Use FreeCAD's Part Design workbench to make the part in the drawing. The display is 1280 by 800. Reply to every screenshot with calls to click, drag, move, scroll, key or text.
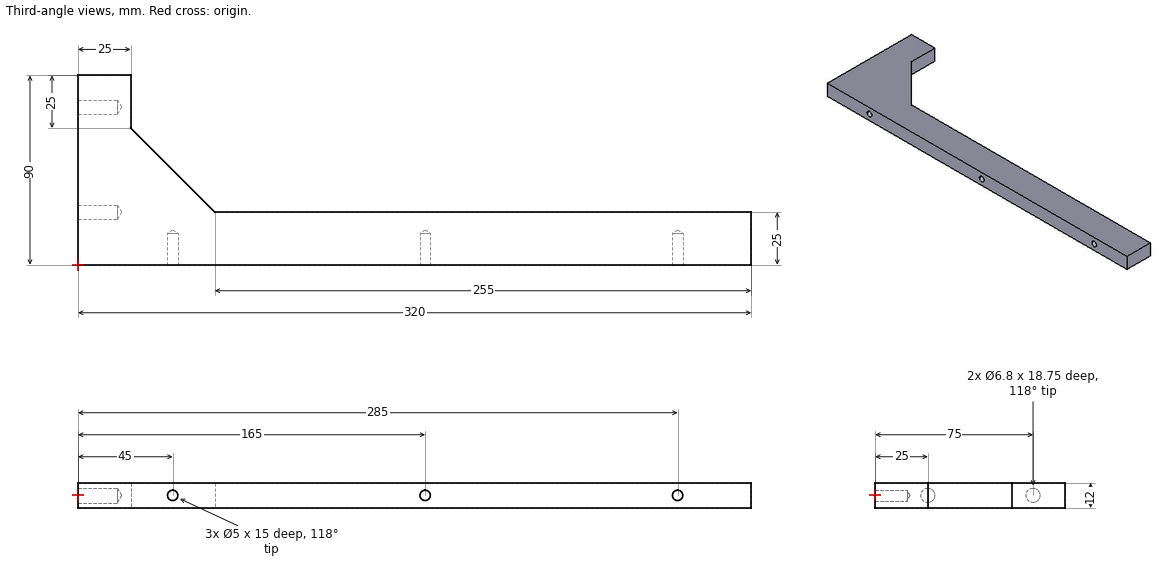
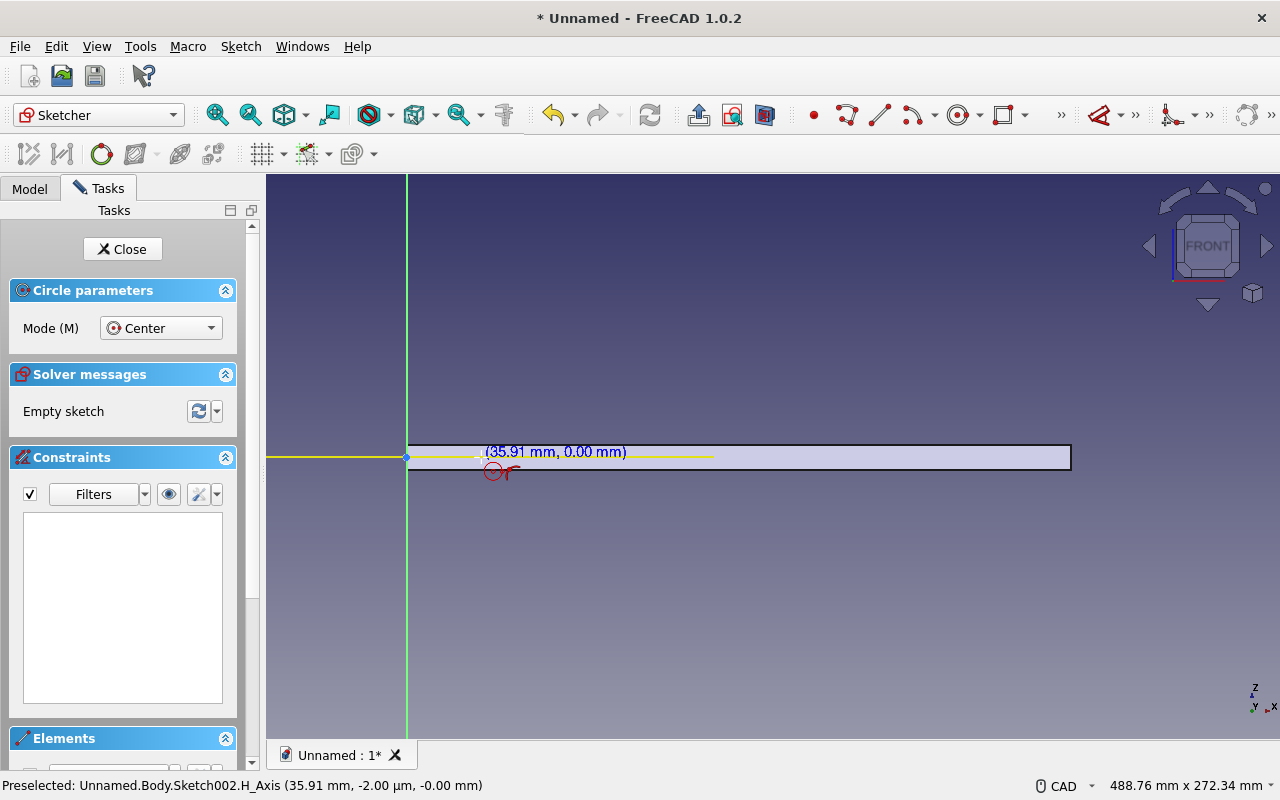
click(500, 457)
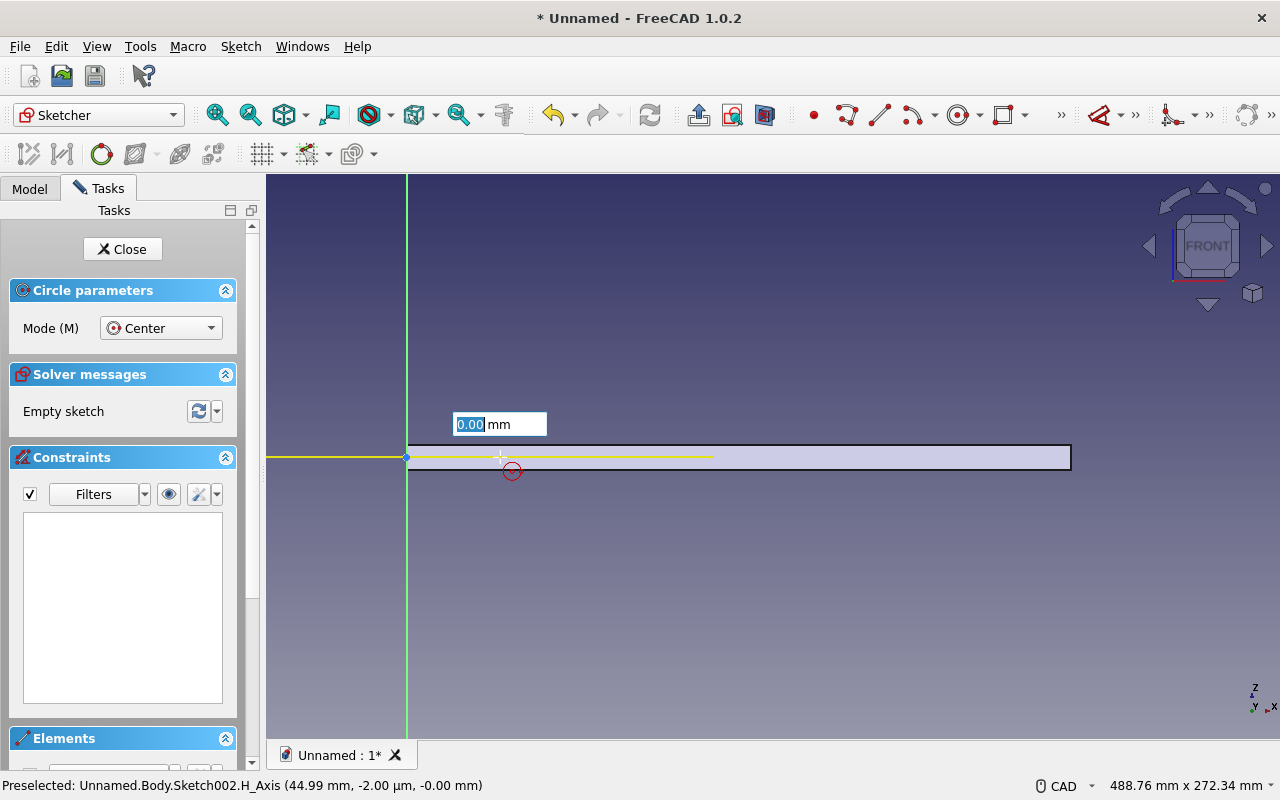
scroll(498, 462, up, 6)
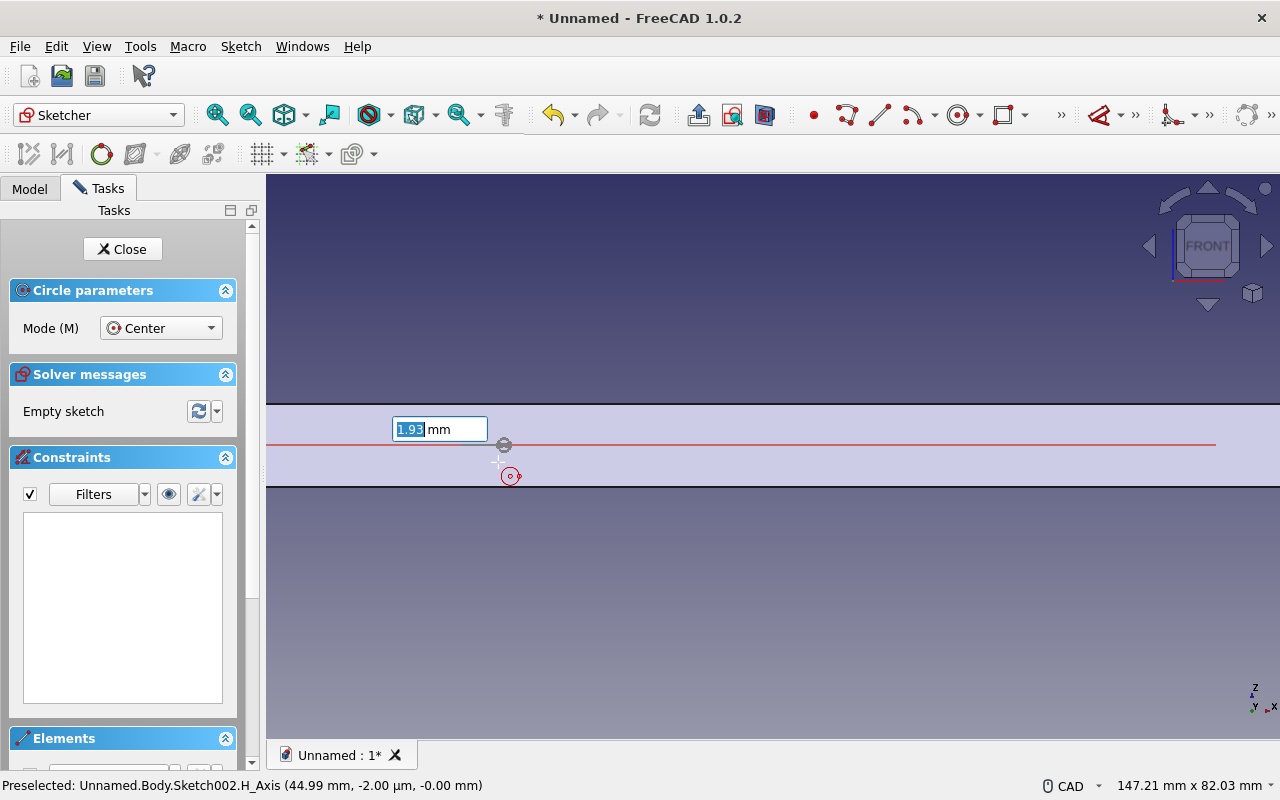
click(498, 461)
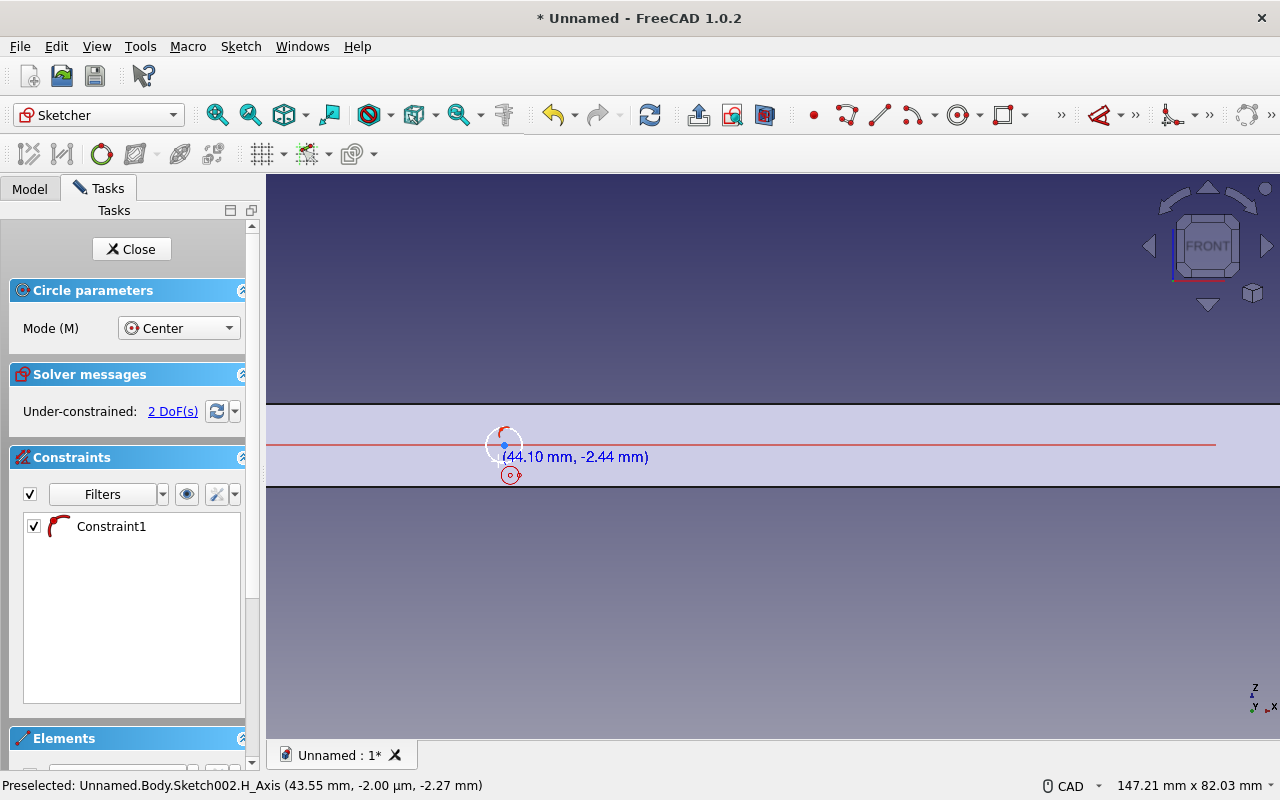
scroll(498, 461, down, 6)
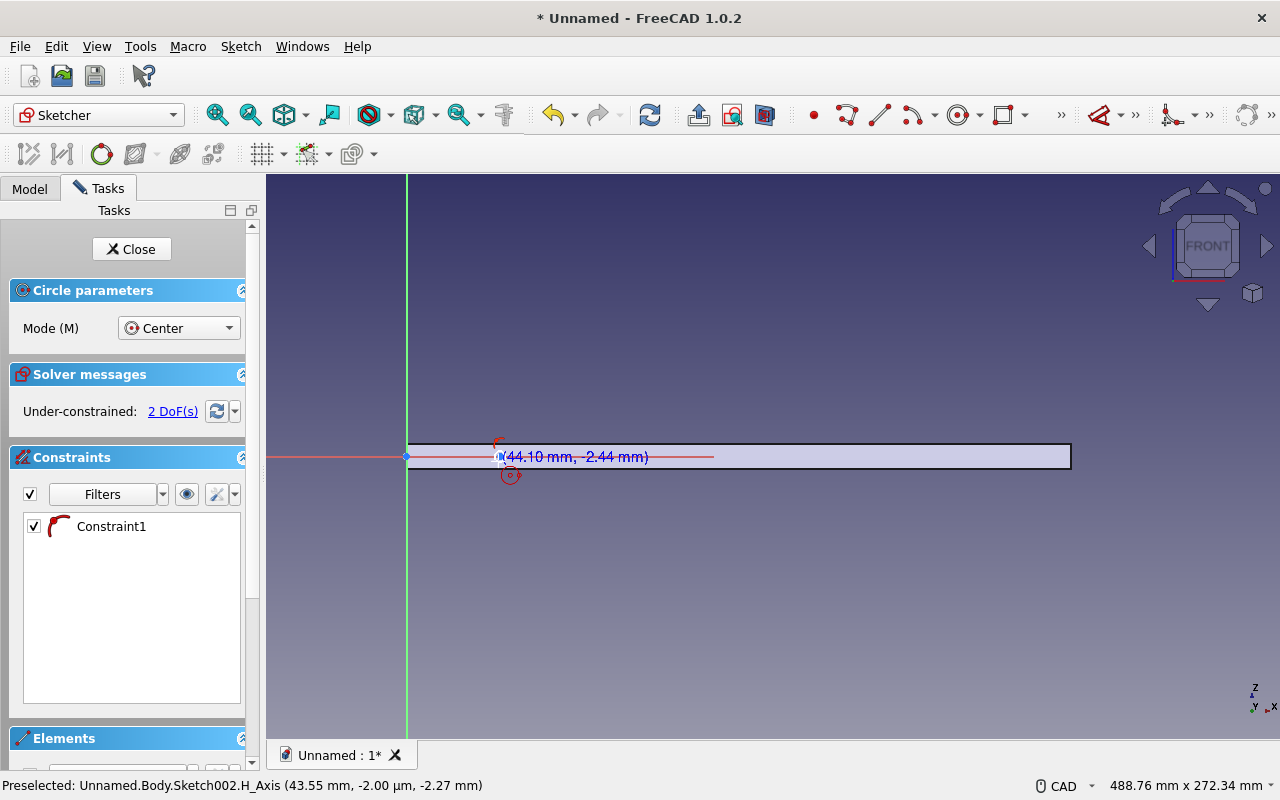
scroll(749, 457, up, 8)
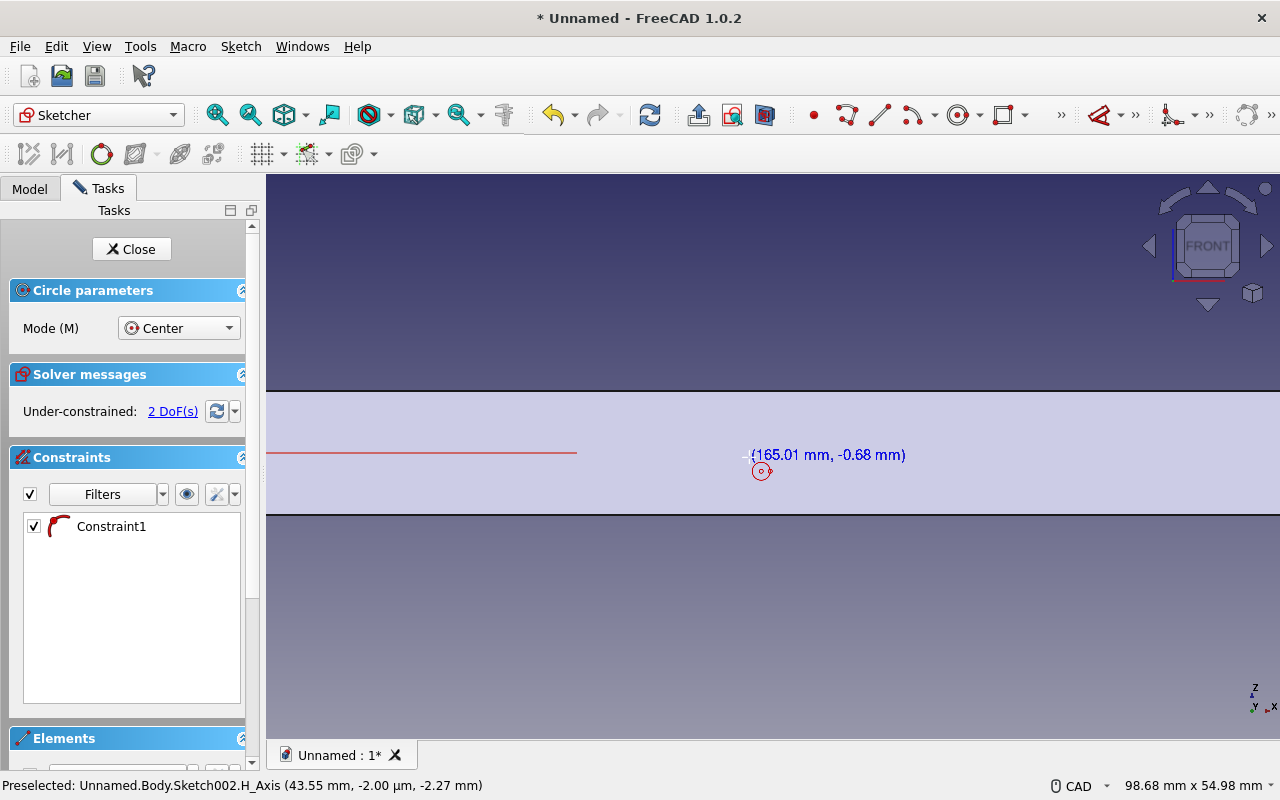
scroll(749, 457, down, 8)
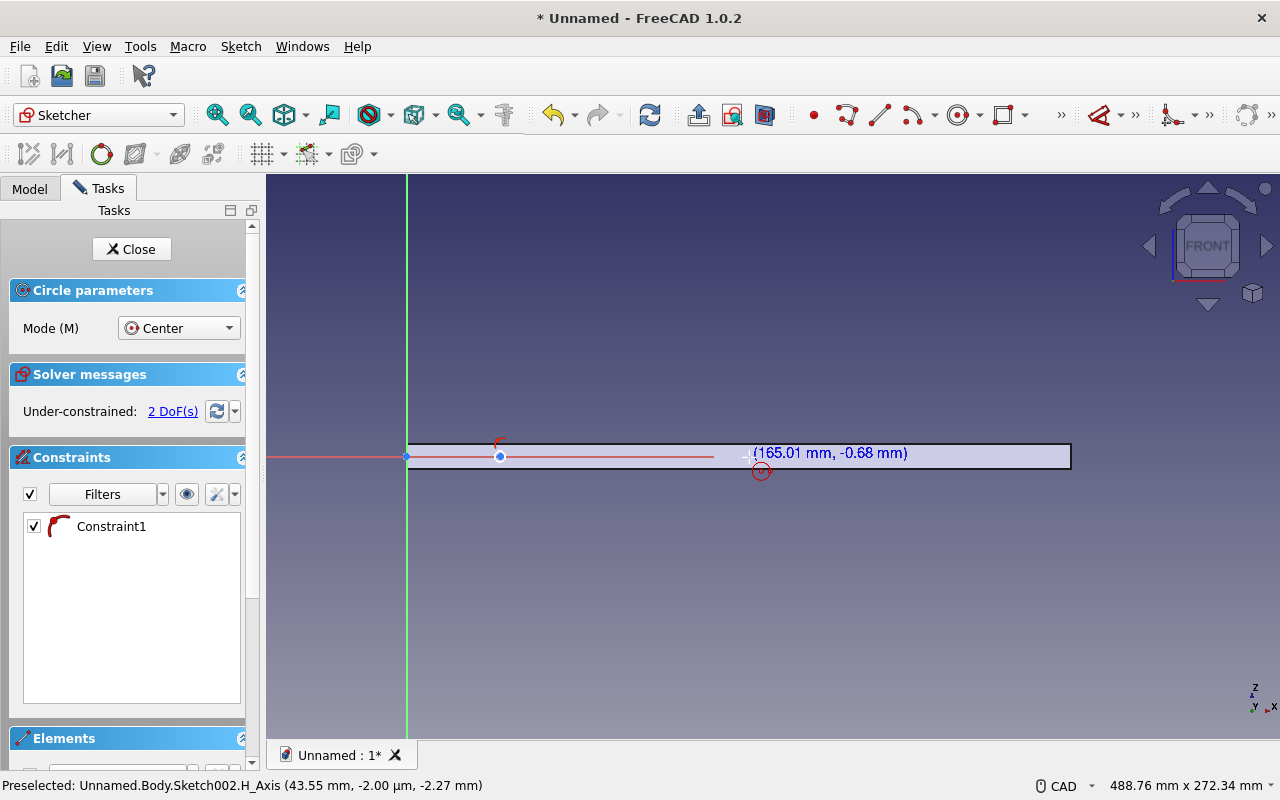
click(749, 457)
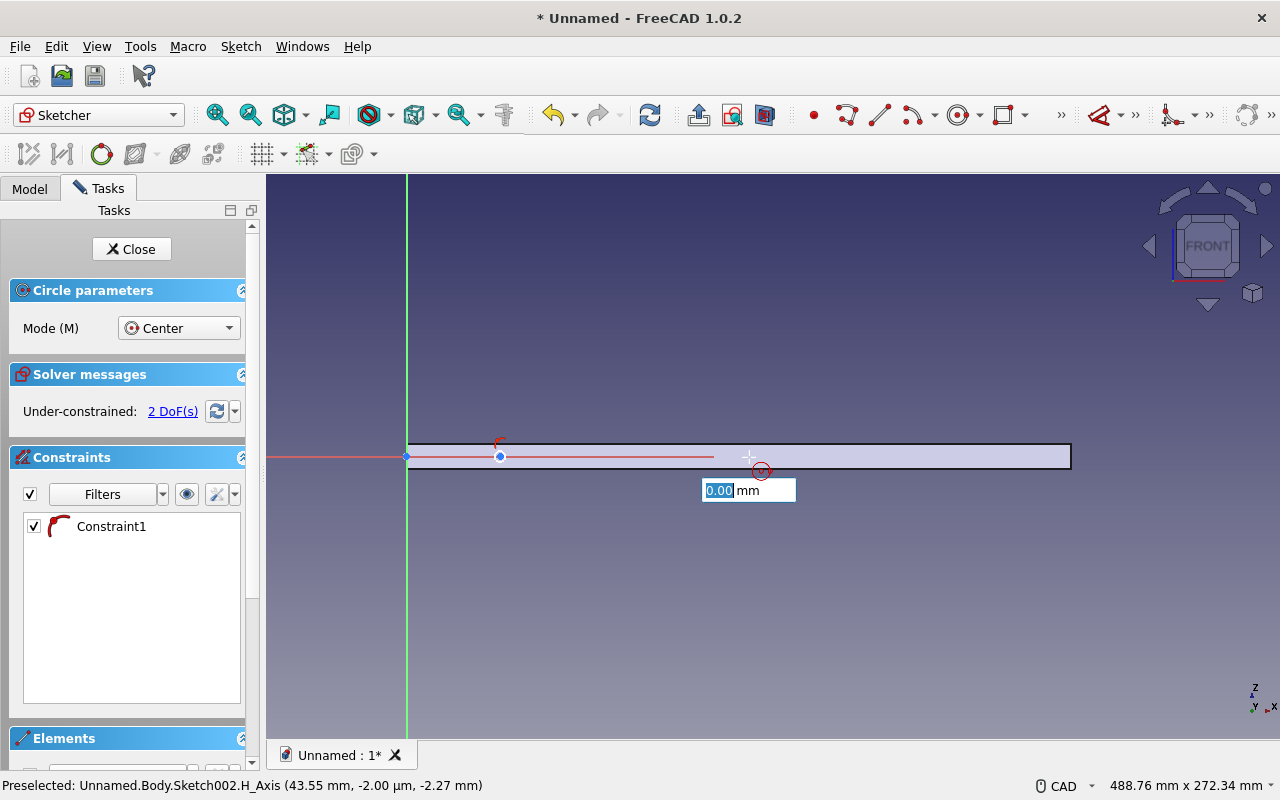
scroll(747, 461, up, 6)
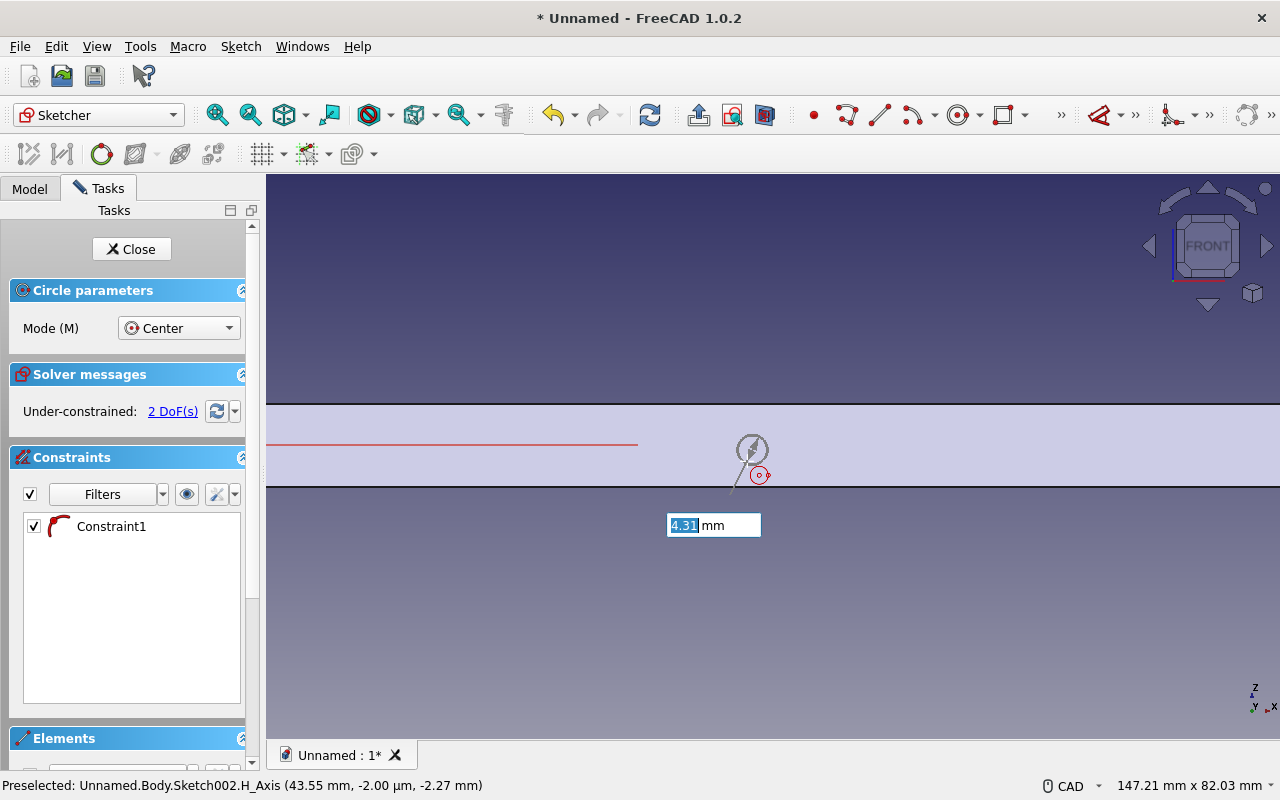
click(747, 461)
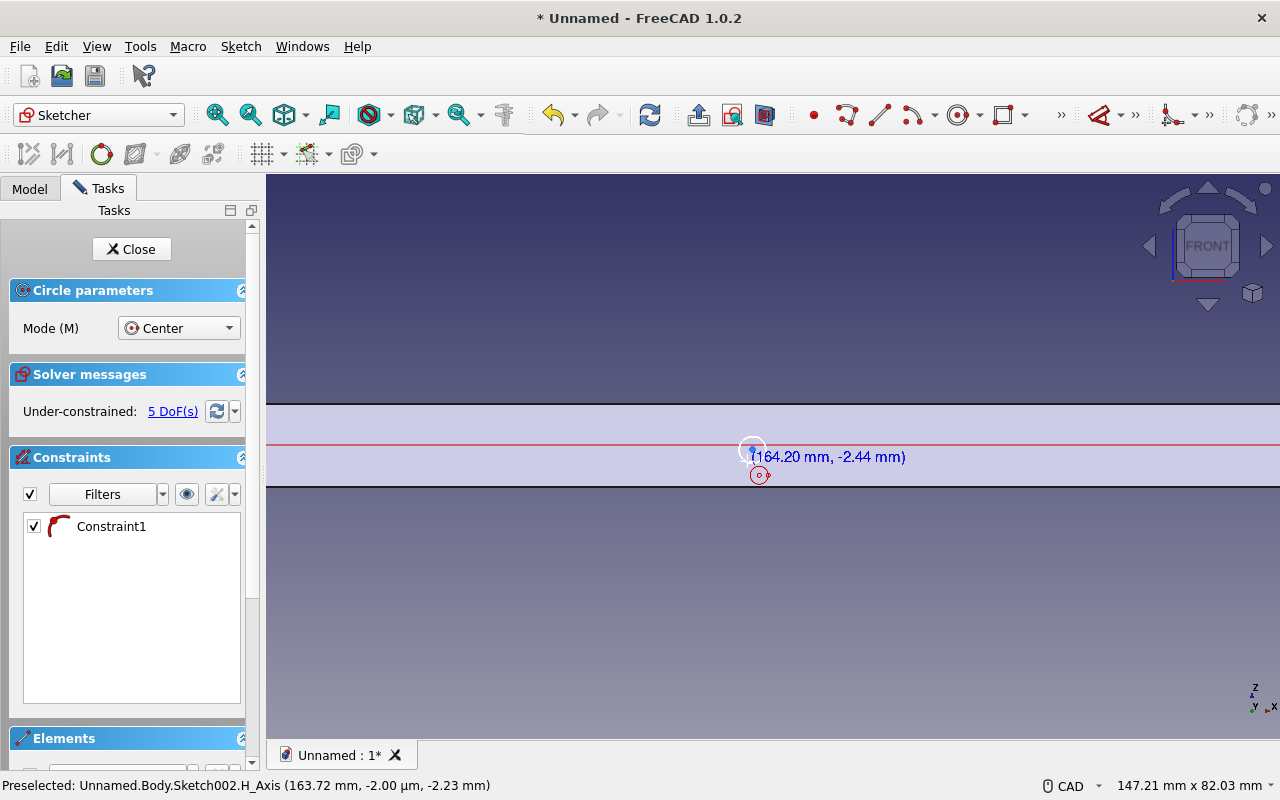
scroll(747, 461, down, 6)